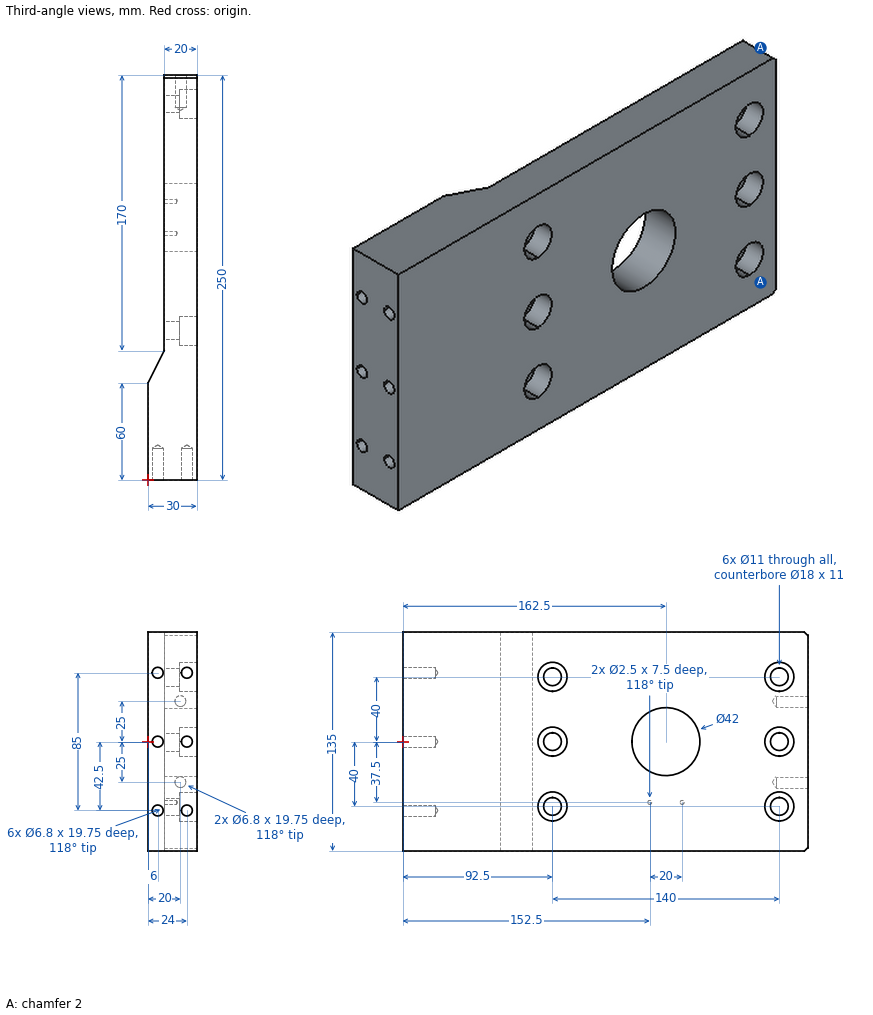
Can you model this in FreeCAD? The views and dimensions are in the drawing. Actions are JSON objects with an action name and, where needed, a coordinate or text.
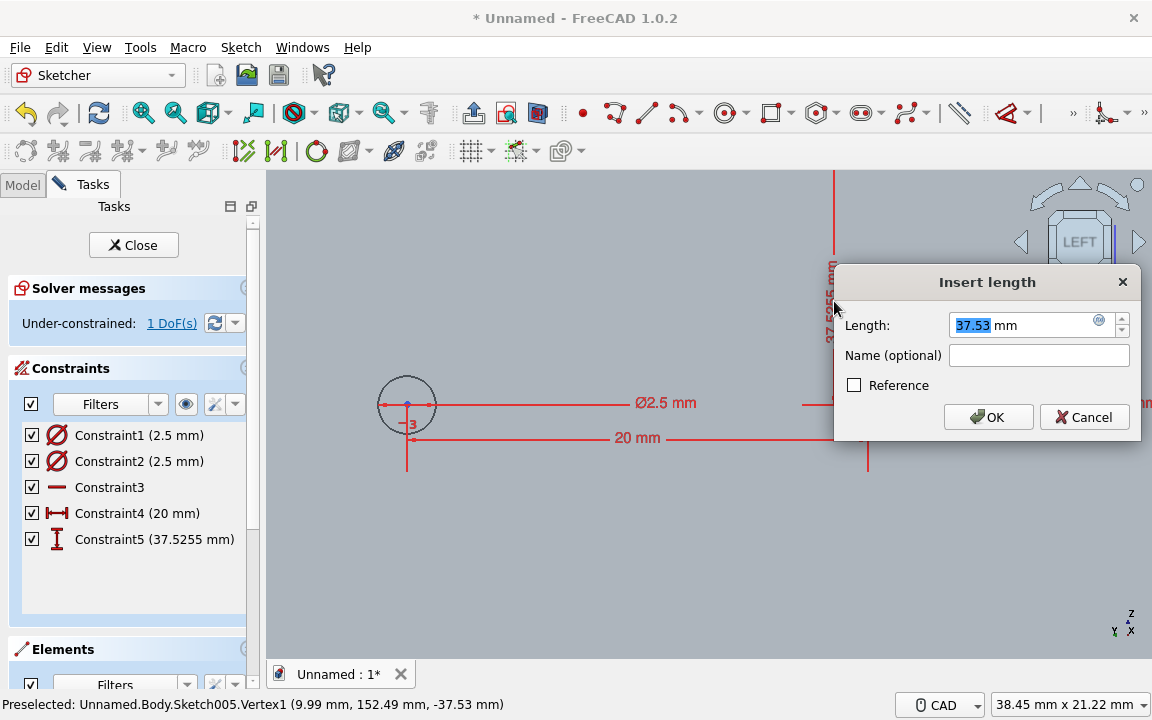
{"action": "type", "text": "37.5"}
{"action": "key", "text": "Return"}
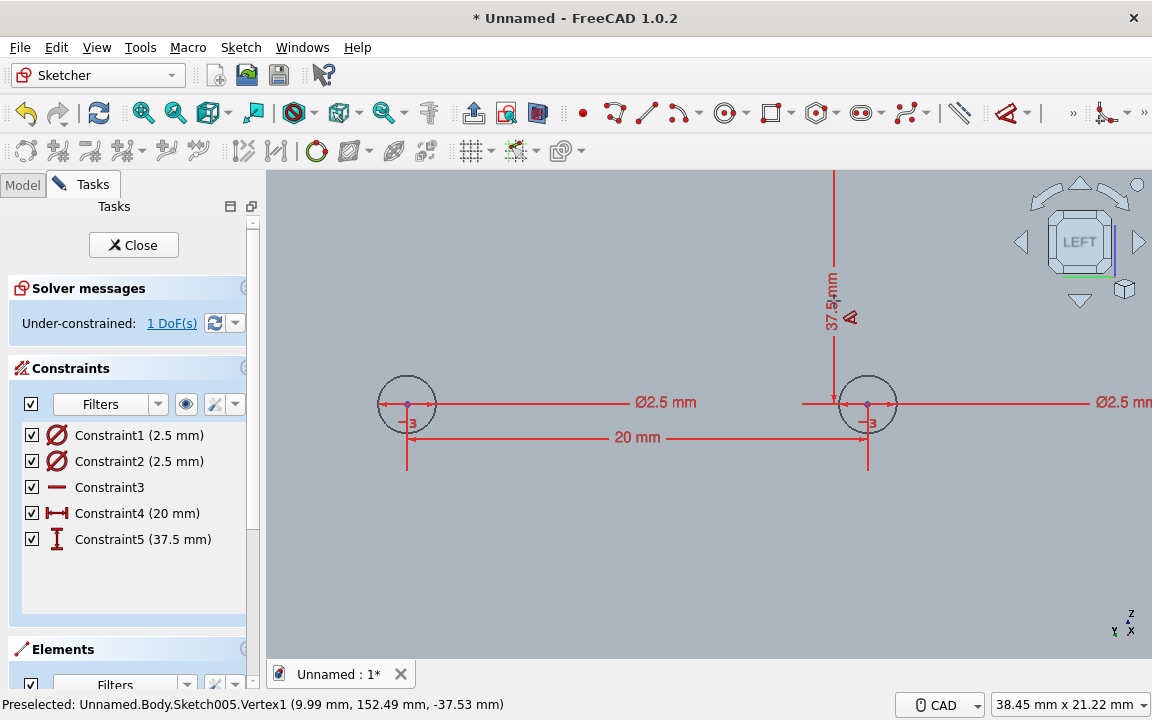
{"action": "left_click", "coordinate": [868, 404]}
{"action": "left_click", "coordinate": [927, 438]}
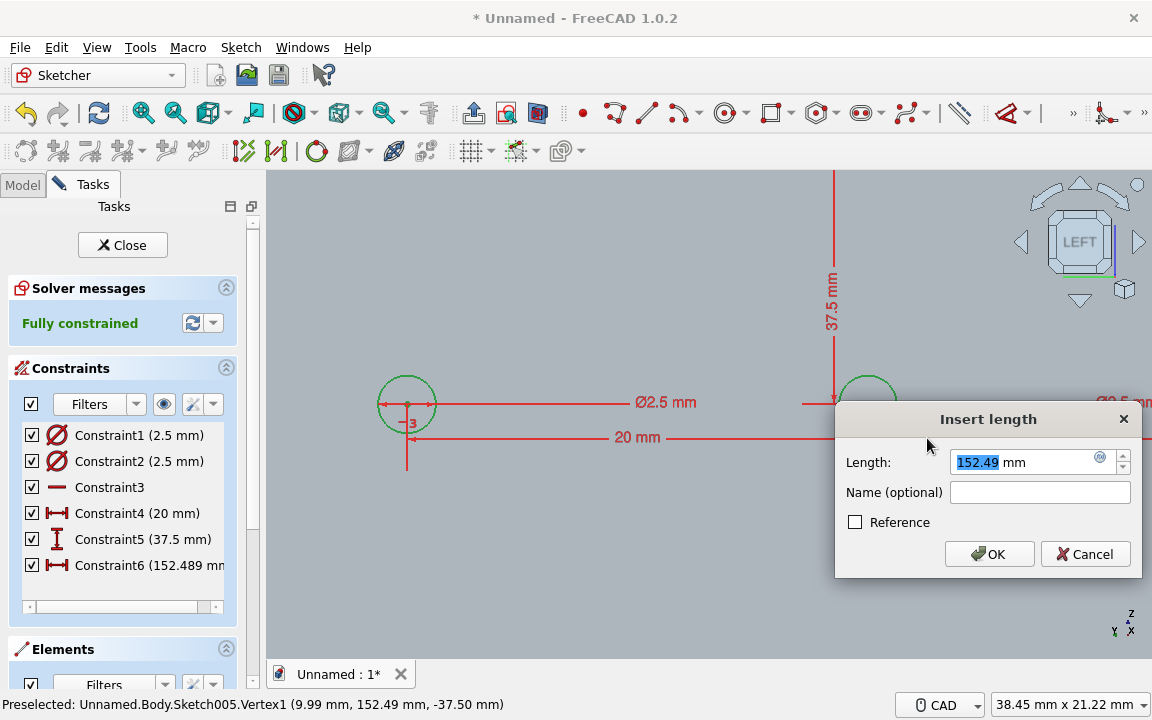
{"action": "type", "text": "152.5"}
{"action": "key", "text": "Return"}
{"action": "key", "text": "Escape"}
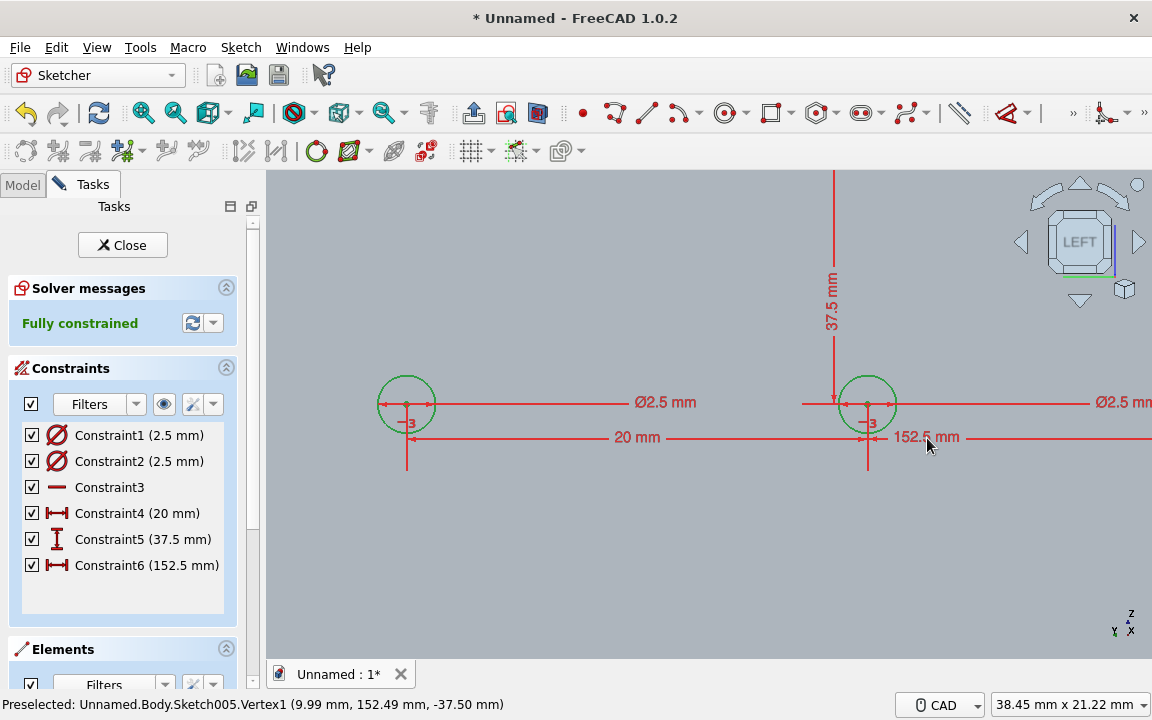
{"action": "left_click", "coordinate": [123, 245]}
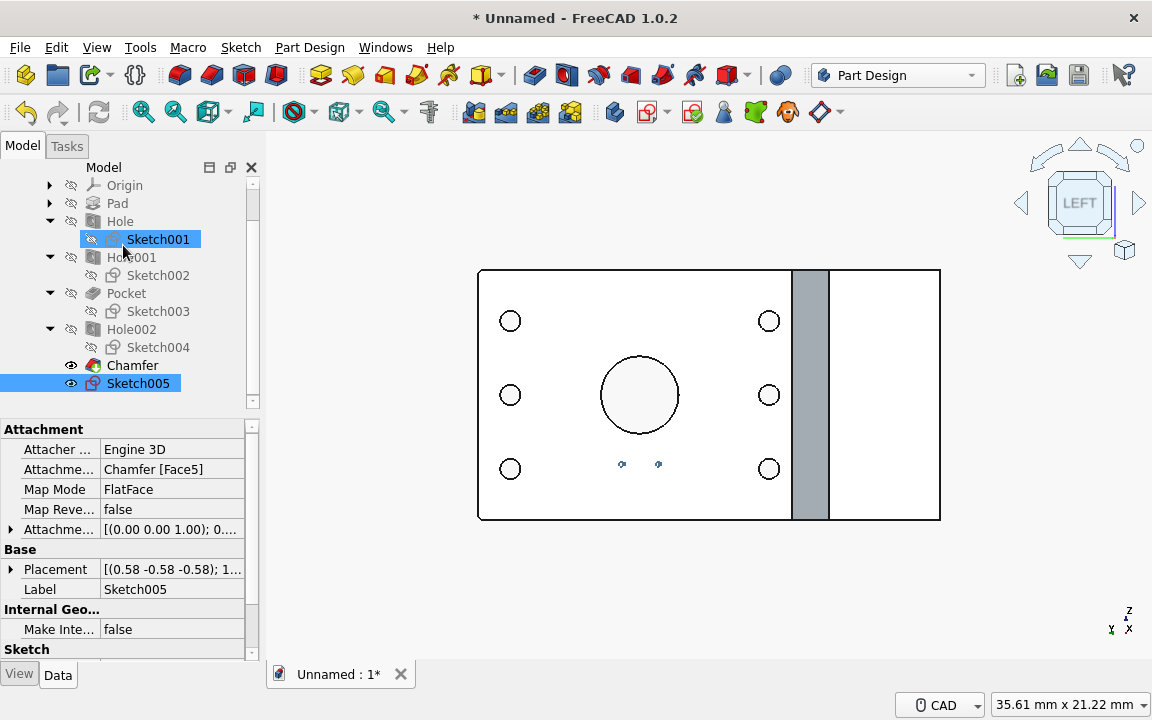
{"action": "left_click", "coordinate": [568, 76]}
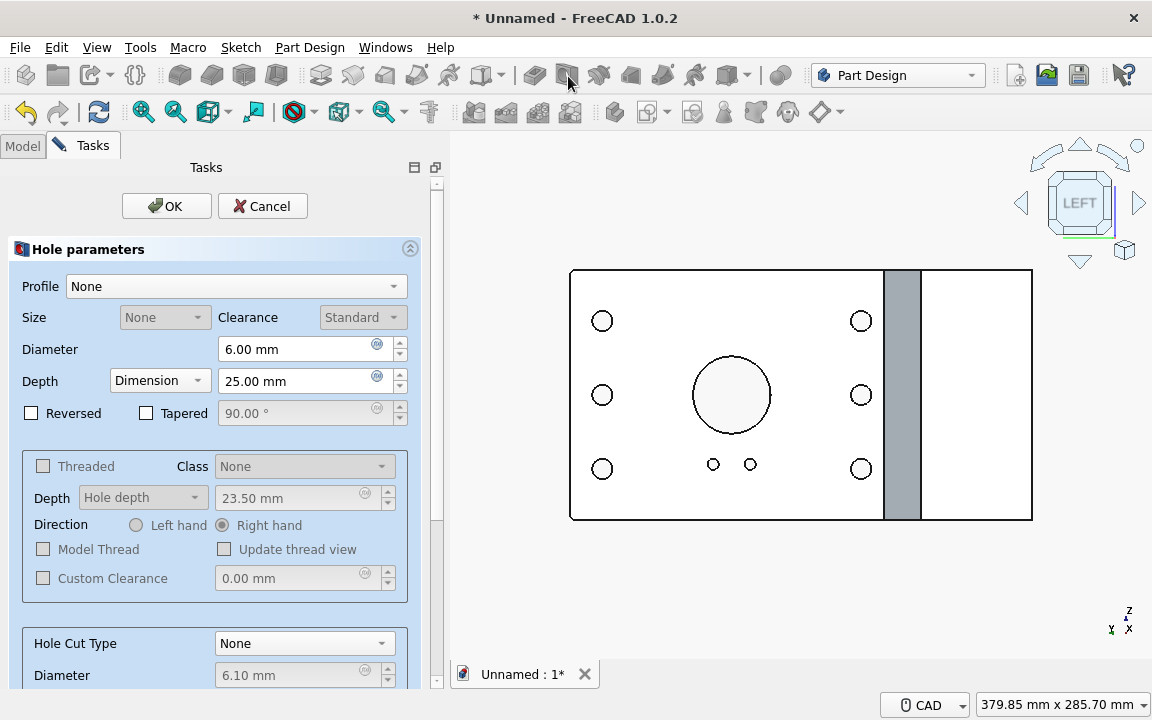
{"action": "triple_click", "coordinate": [305, 349]}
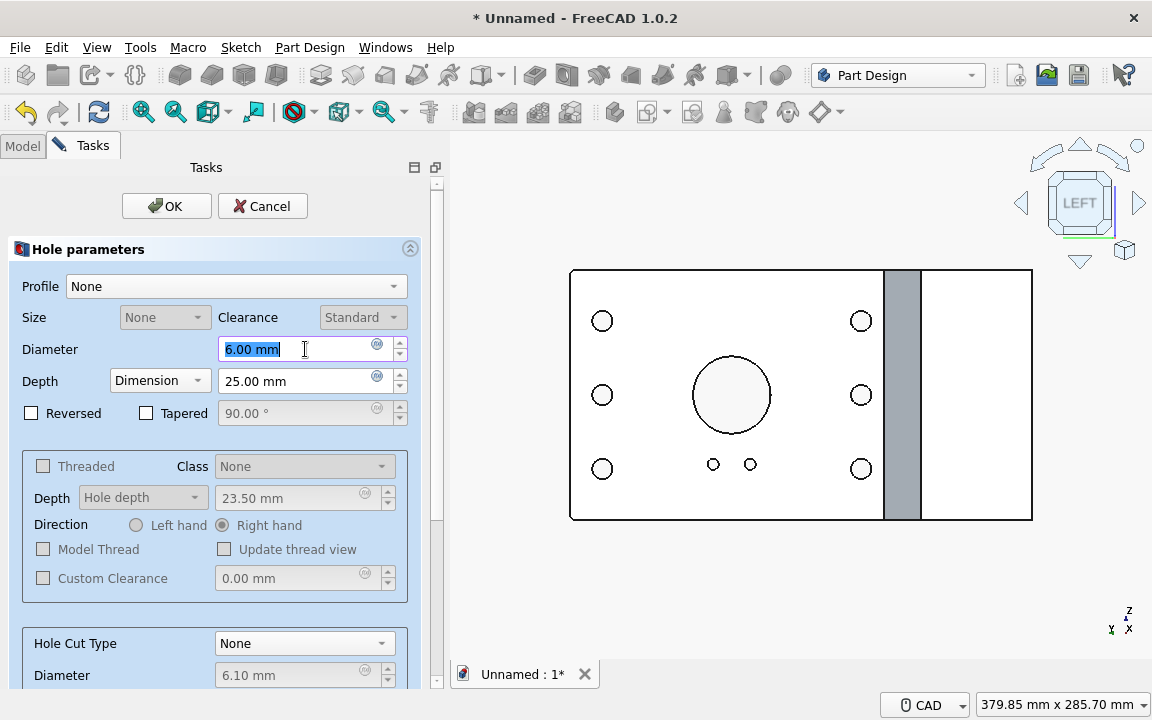
{"action": "type", "text": "2.5"}
{"action": "key", "text": "Tab"}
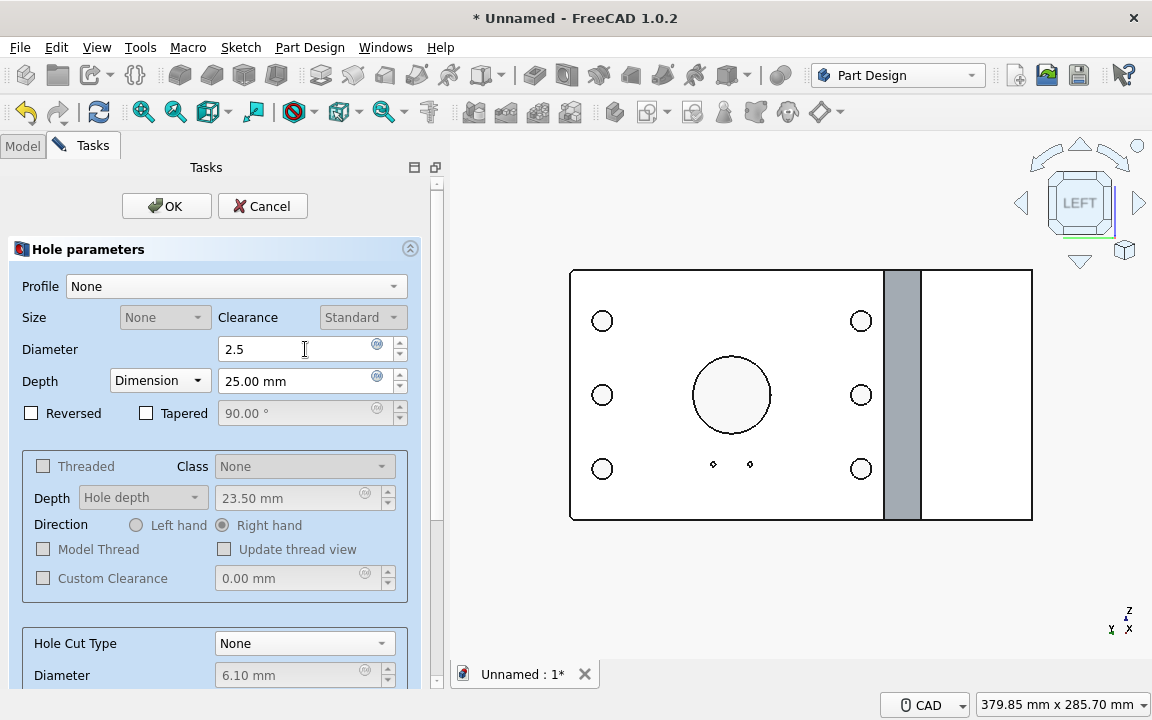
{"action": "triple_click", "coordinate": [305, 381]}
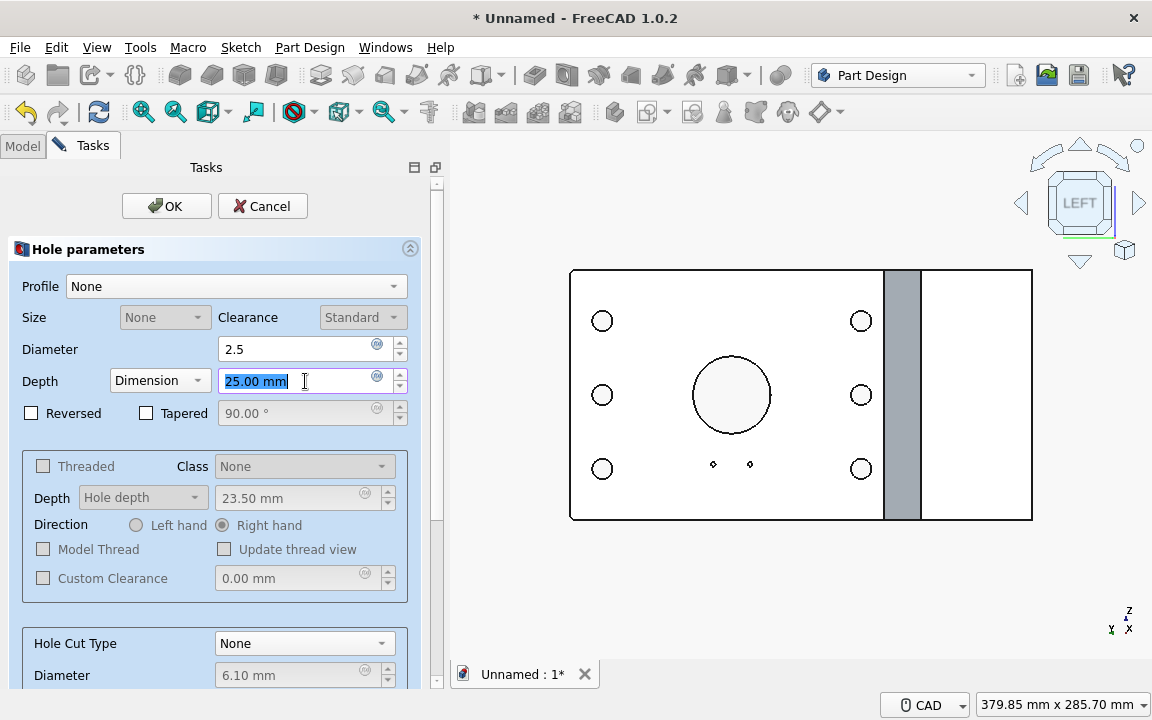
{"action": "type", "text": "7.5"}
{"action": "key", "text": "Tab"}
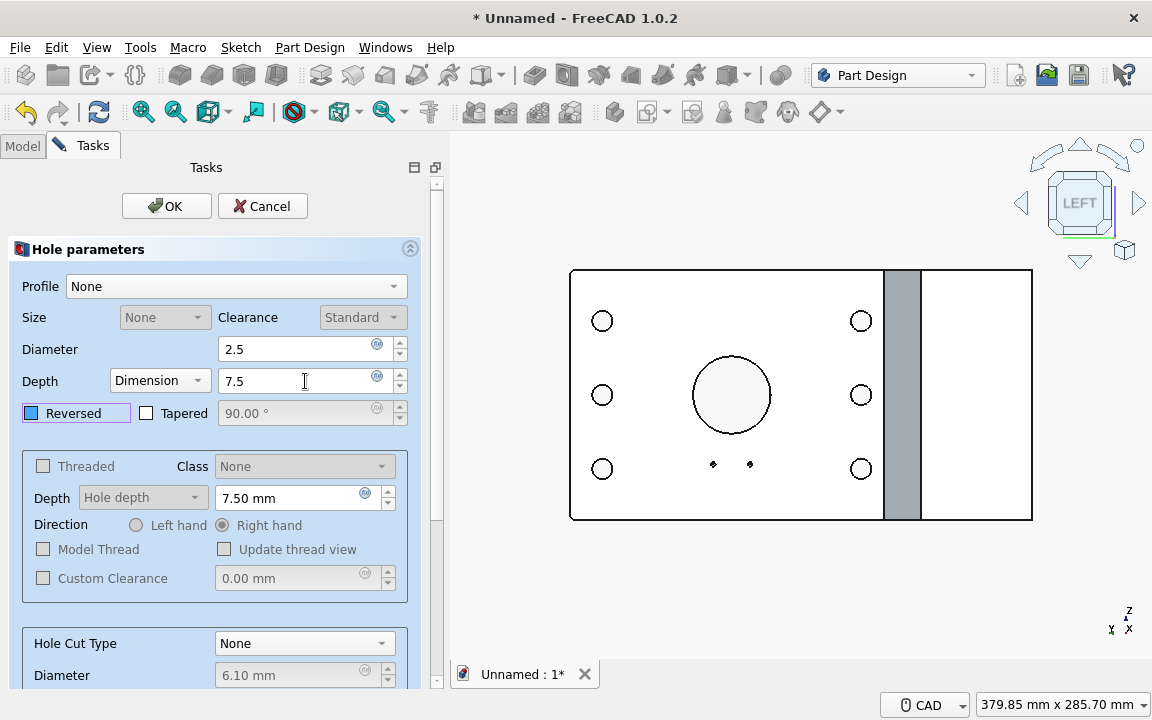
{"action": "left_click", "coordinate": [167, 206]}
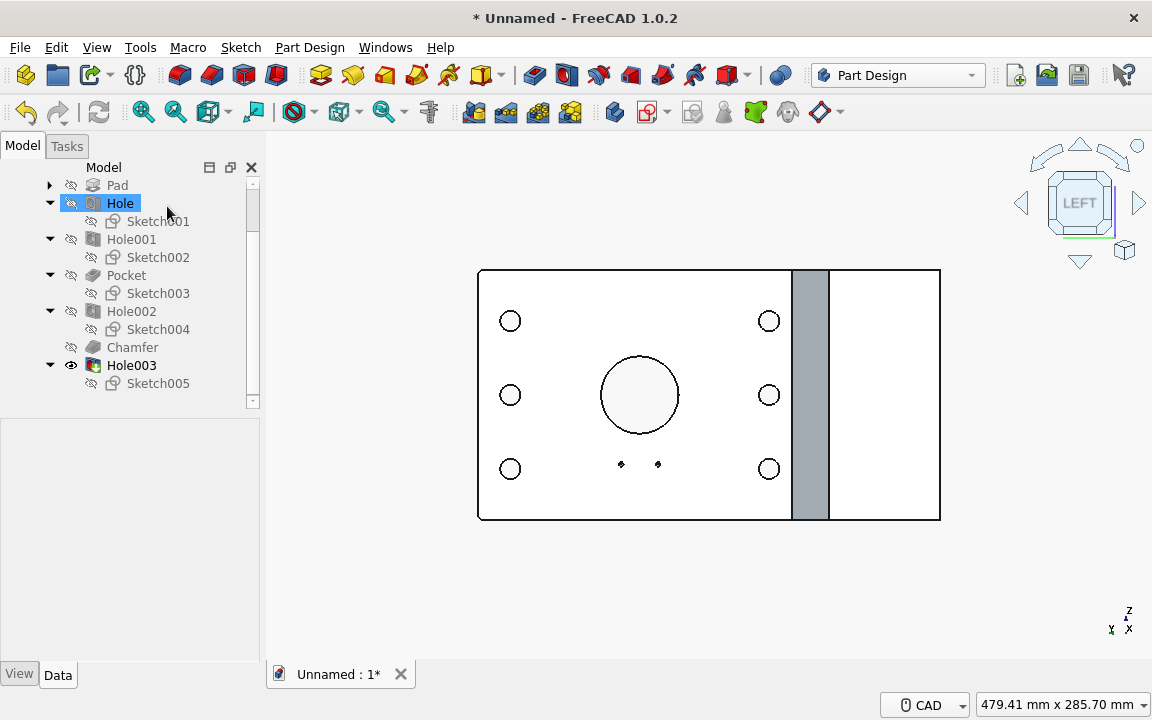
{"action": "key", "text": "0"}